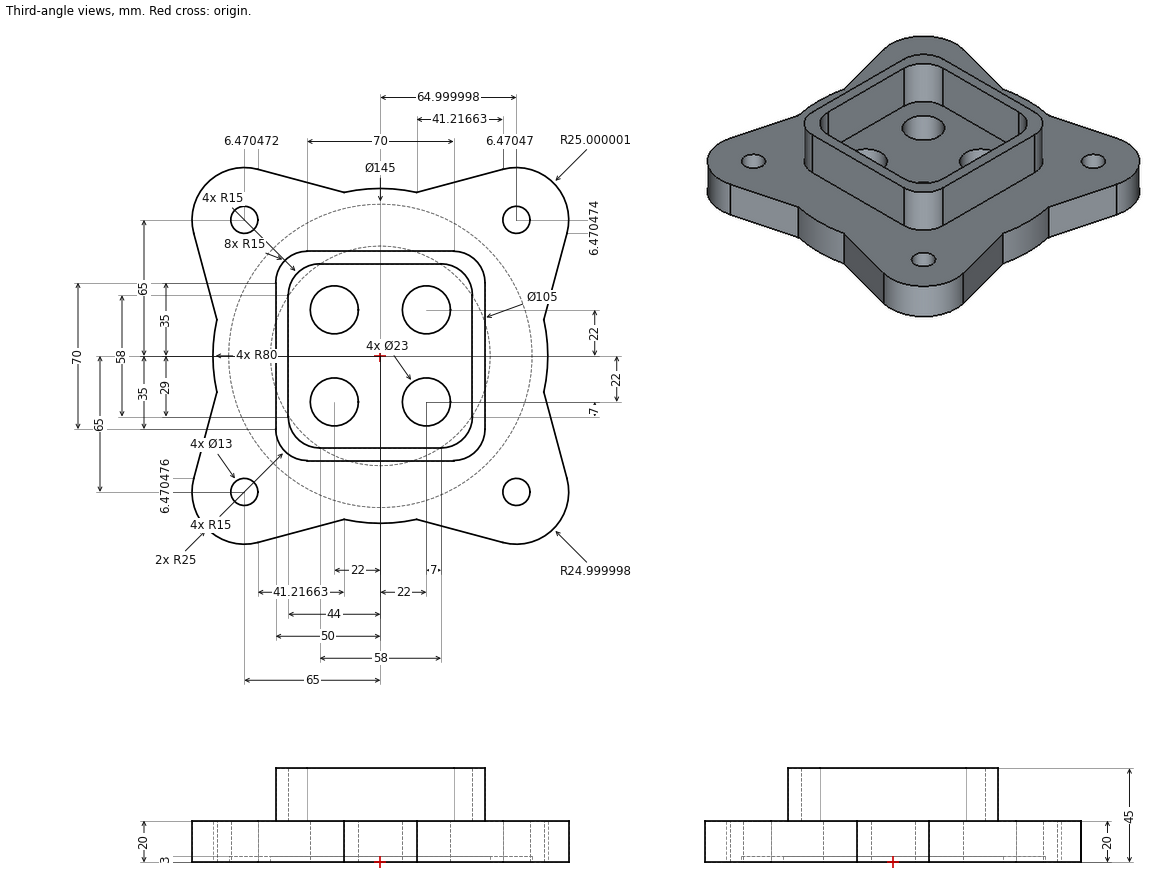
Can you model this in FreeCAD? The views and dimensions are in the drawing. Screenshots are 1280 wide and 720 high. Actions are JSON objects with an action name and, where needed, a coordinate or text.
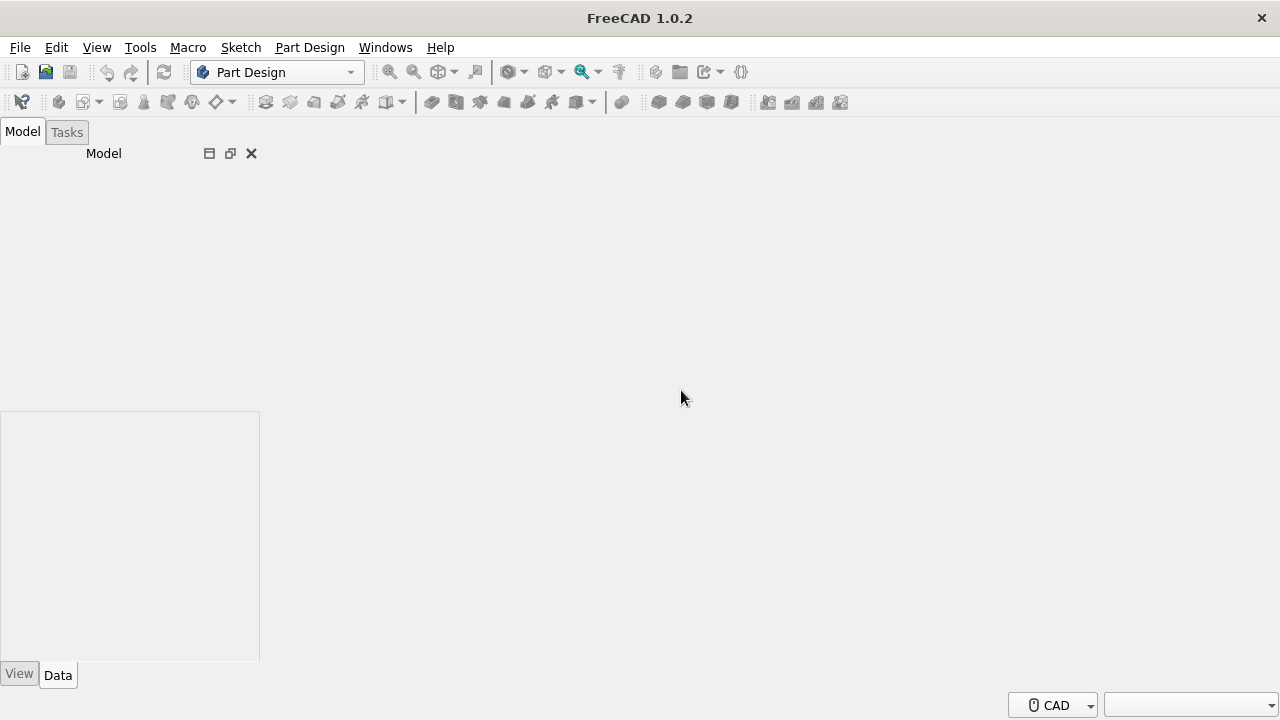
{"action": "left_click", "coordinate": [22, 72]}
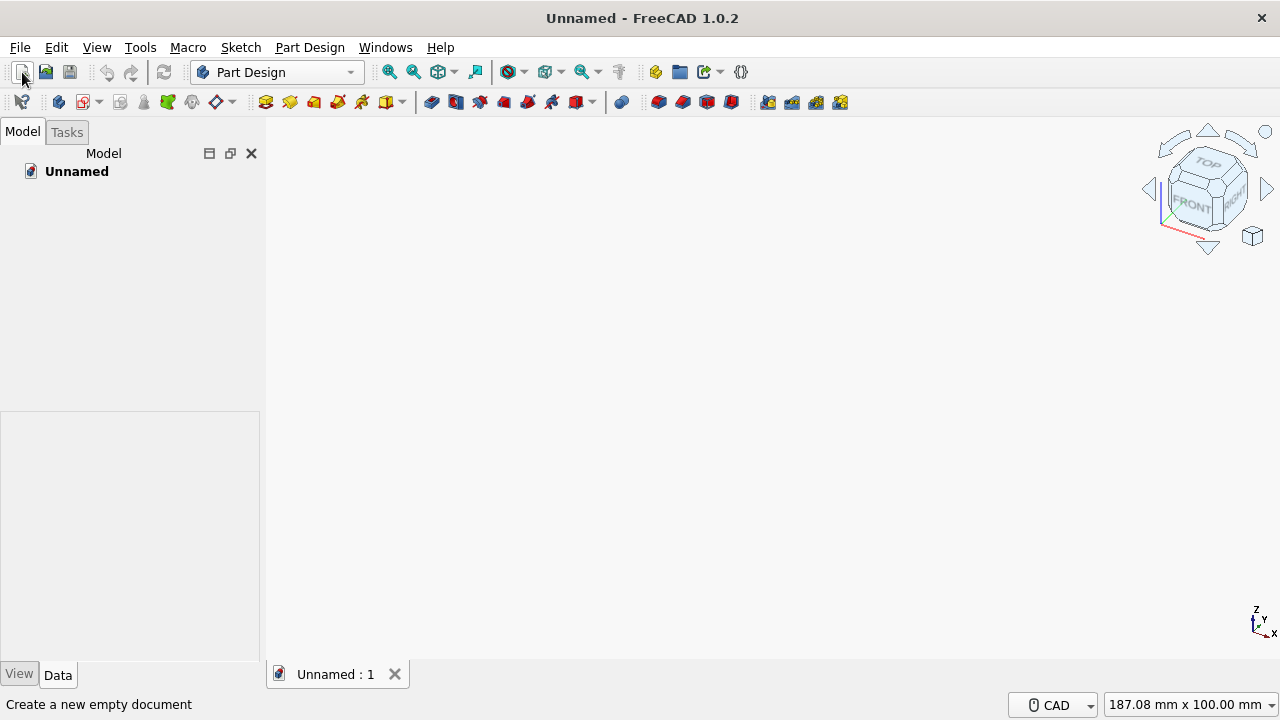
{"action": "left_click", "coordinate": [84, 102]}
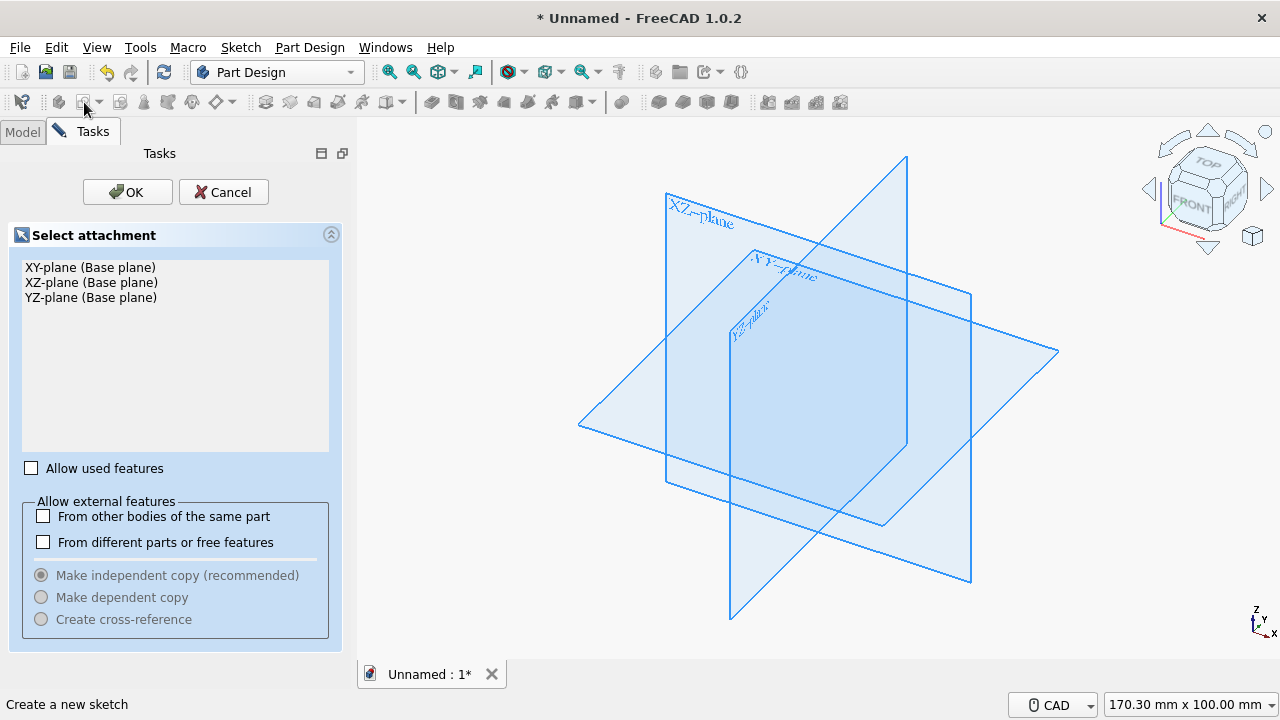
{"action": "left_click", "coordinate": [82, 268]}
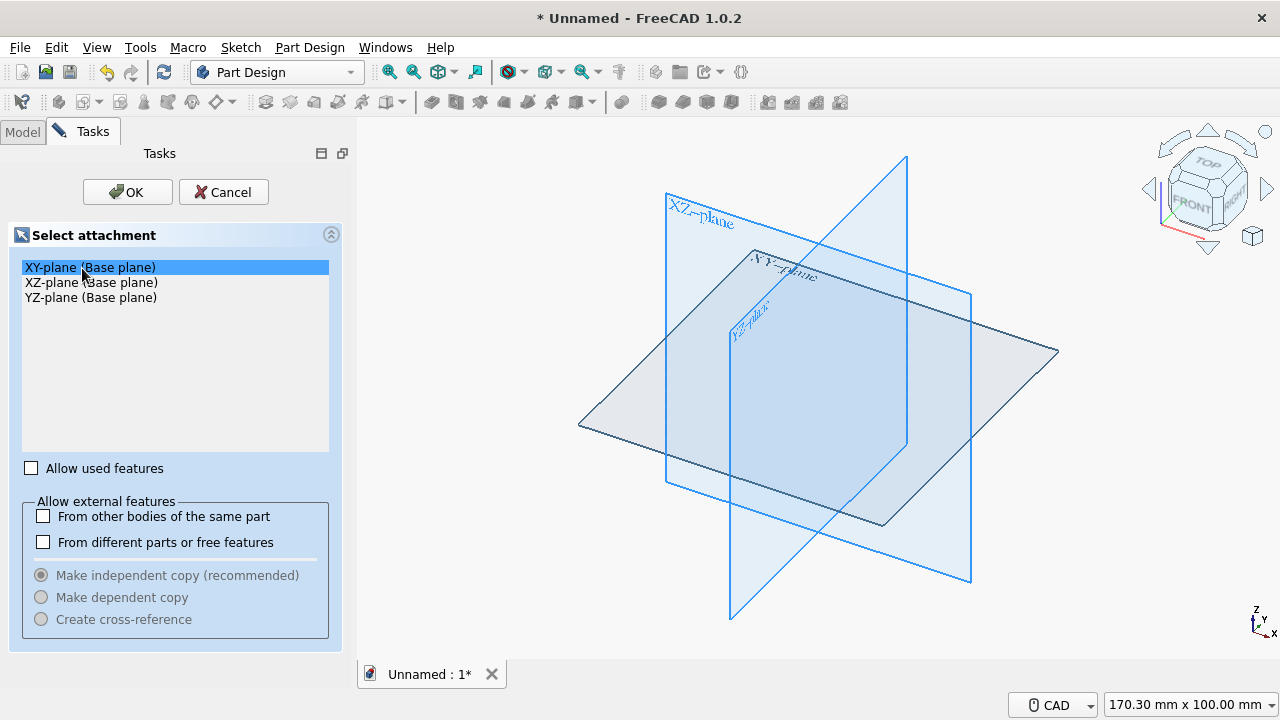
{"action": "left_click", "coordinate": [128, 192]}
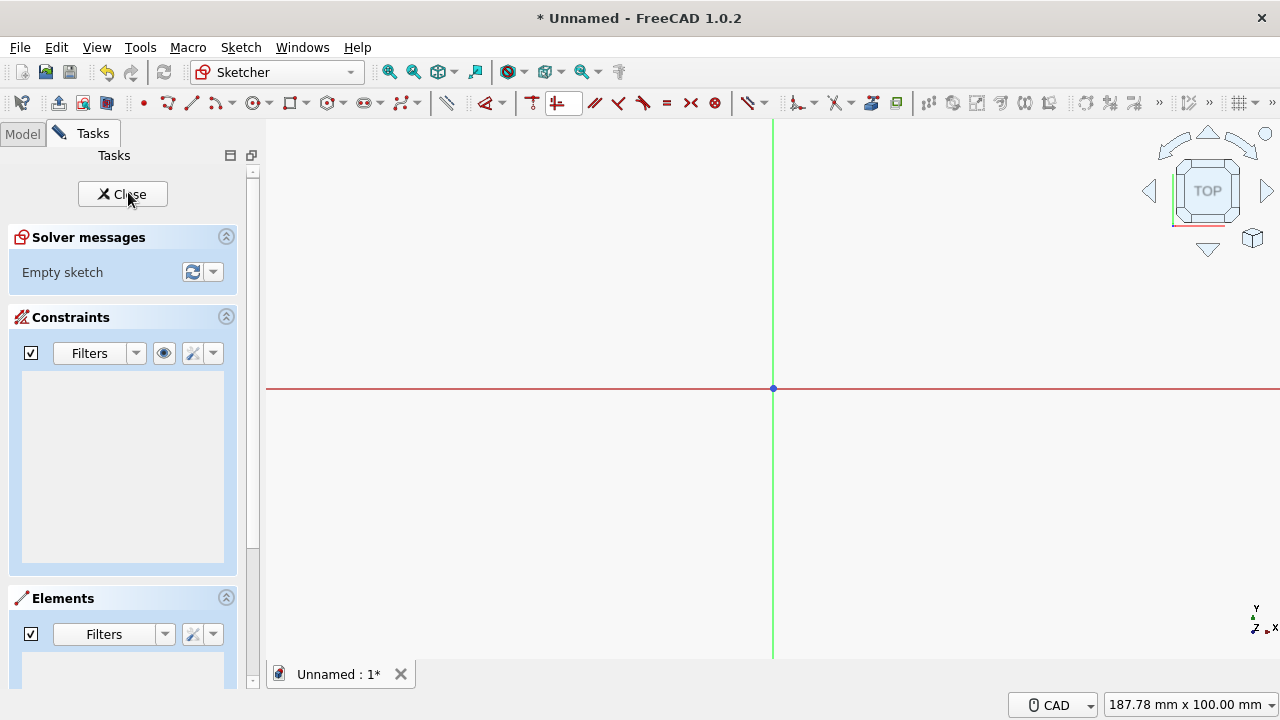
{"action": "scroll", "coordinate": [665, 389], "scroll_direction": "down", "scroll_amount": 5}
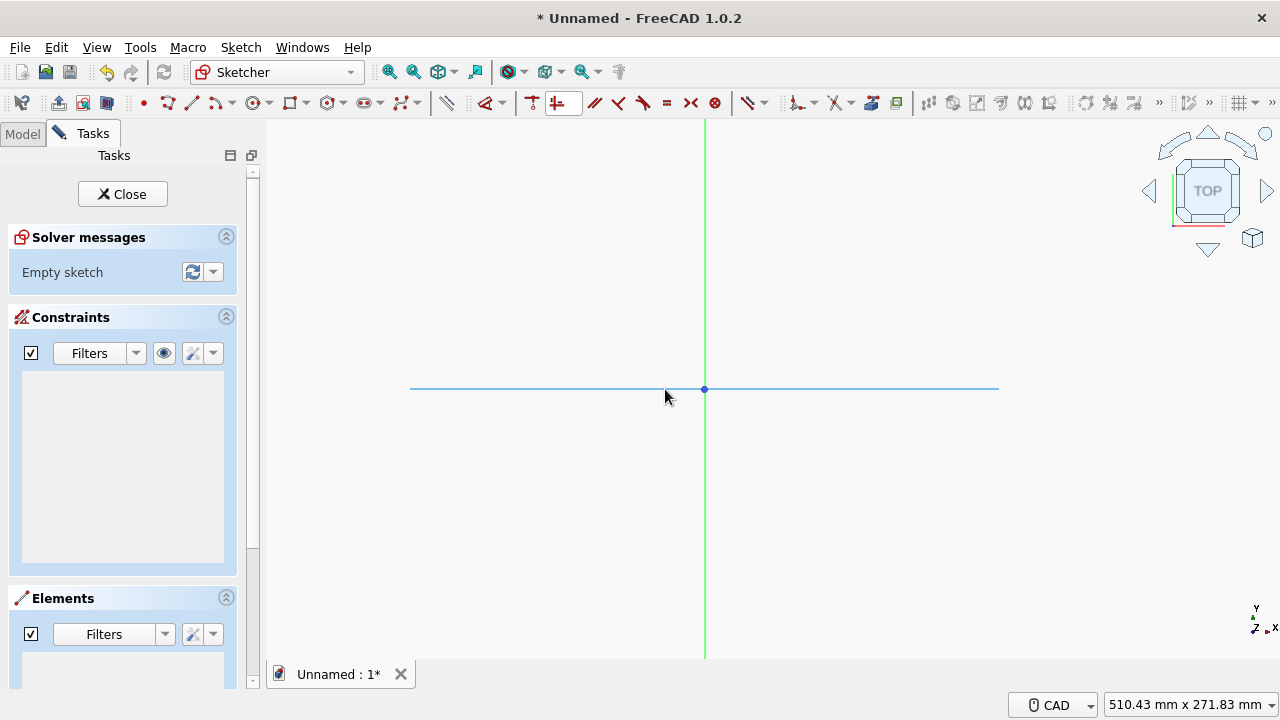
{"action": "left_click", "coordinate": [192, 104]}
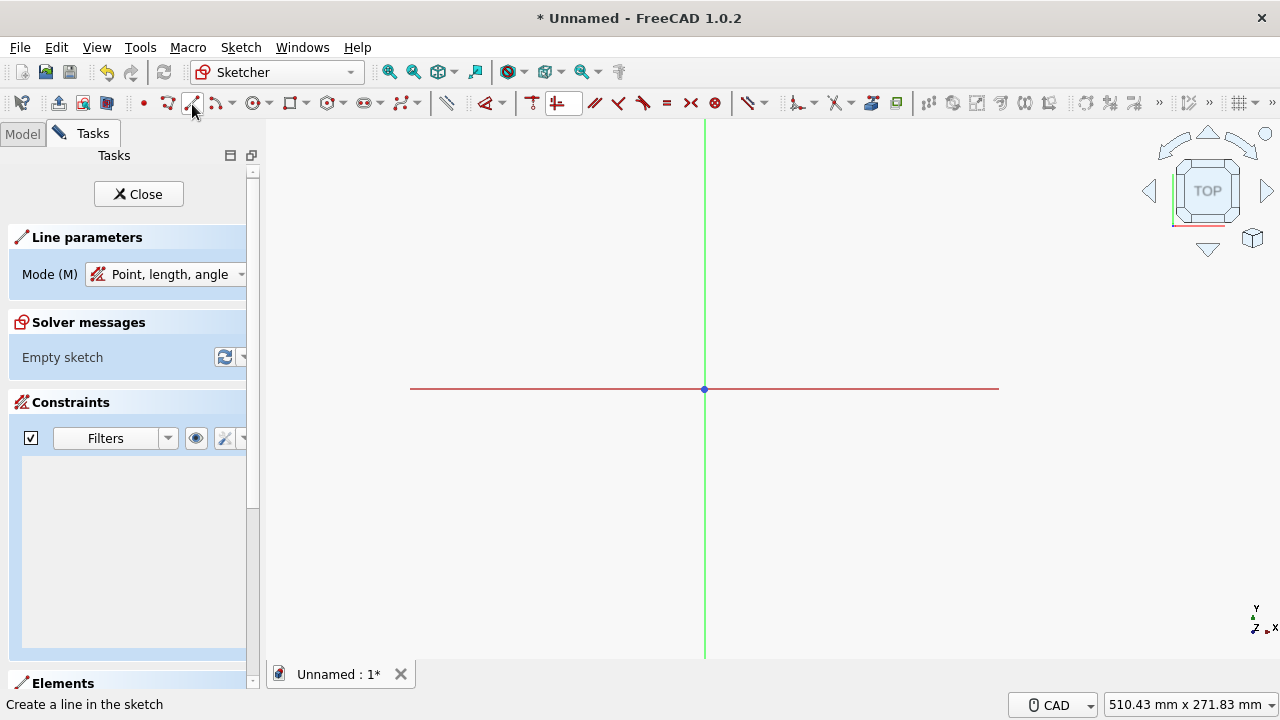
{"action": "left_click", "coordinate": [528, 273]}
{"action": "left_click", "coordinate": [550, 355]}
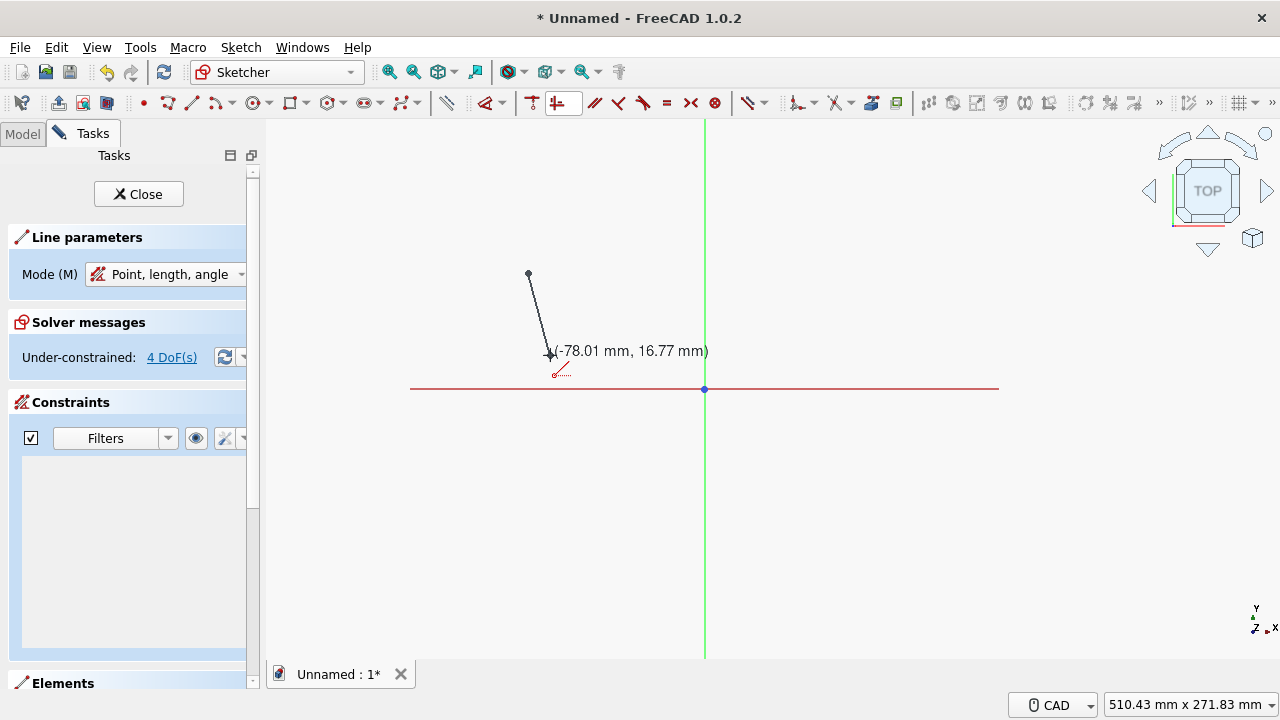
{"action": "left_click", "coordinate": [550, 424]}
{"action": "left_click", "coordinate": [528, 506]}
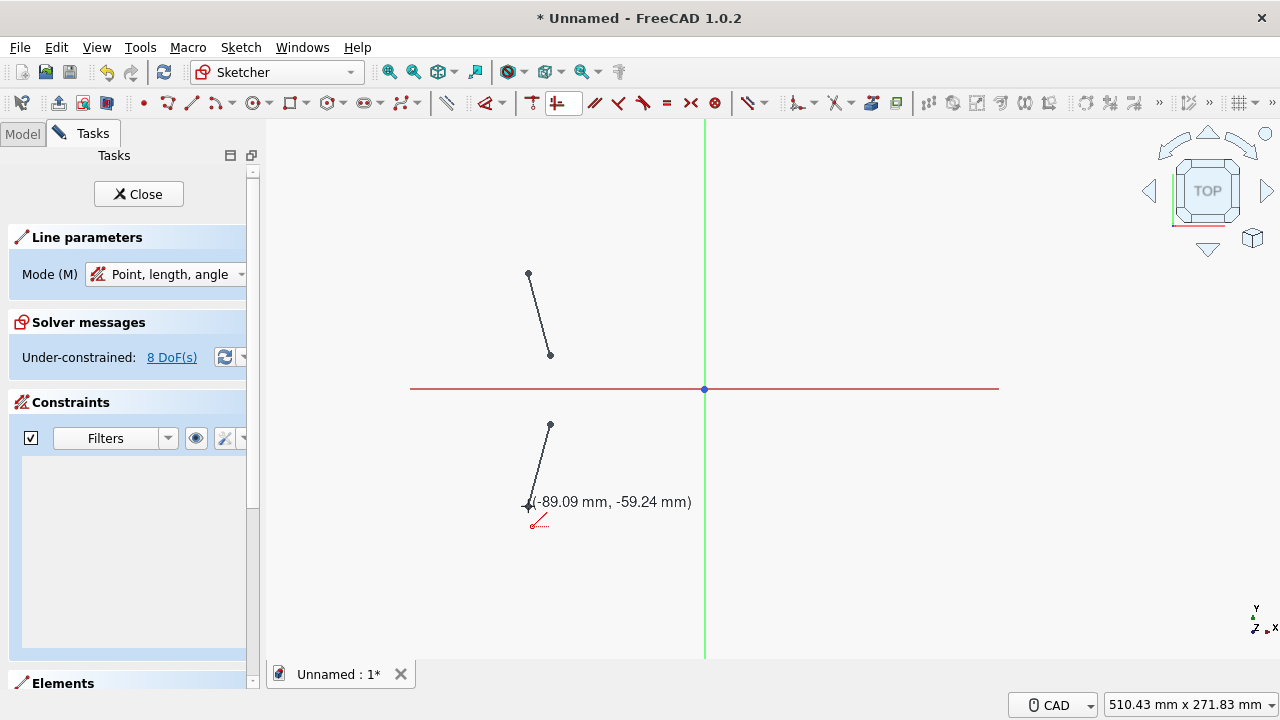
{"action": "left_click", "coordinate": [589, 566]}
{"action": "left_click", "coordinate": [671, 544]}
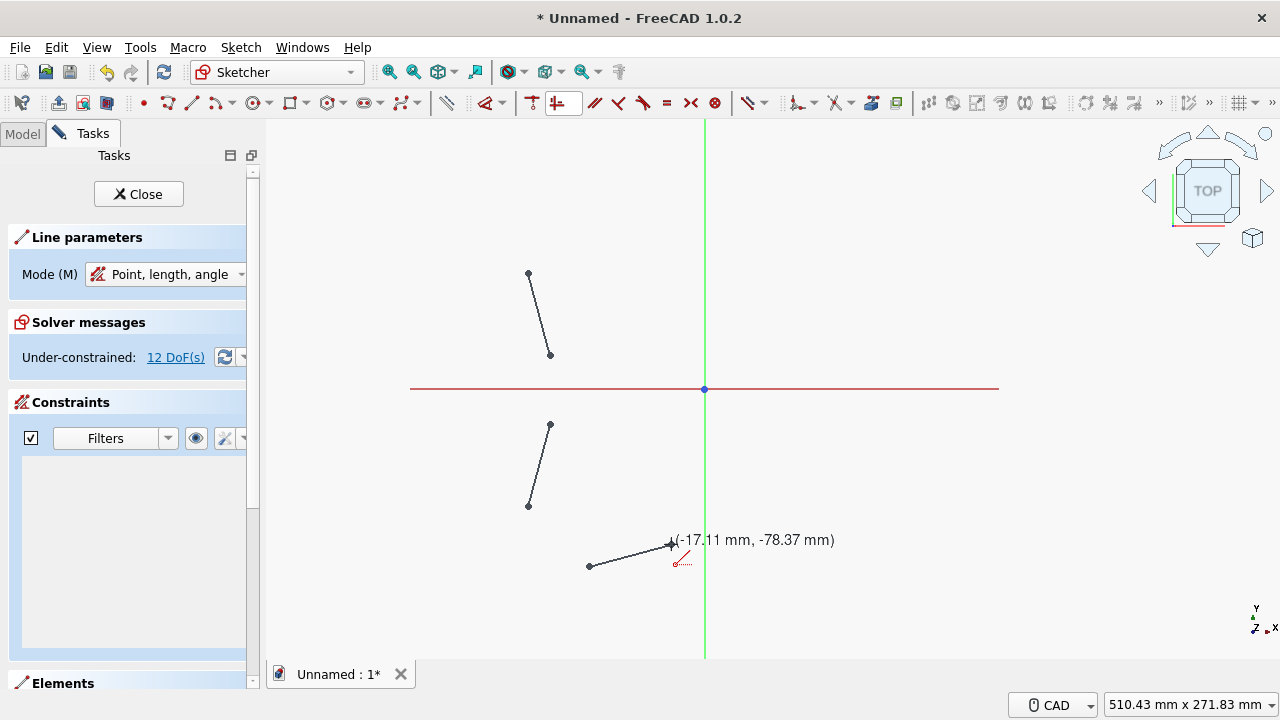
{"action": "left_click", "coordinate": [739, 544]}
{"action": "left_click", "coordinate": [821, 566]}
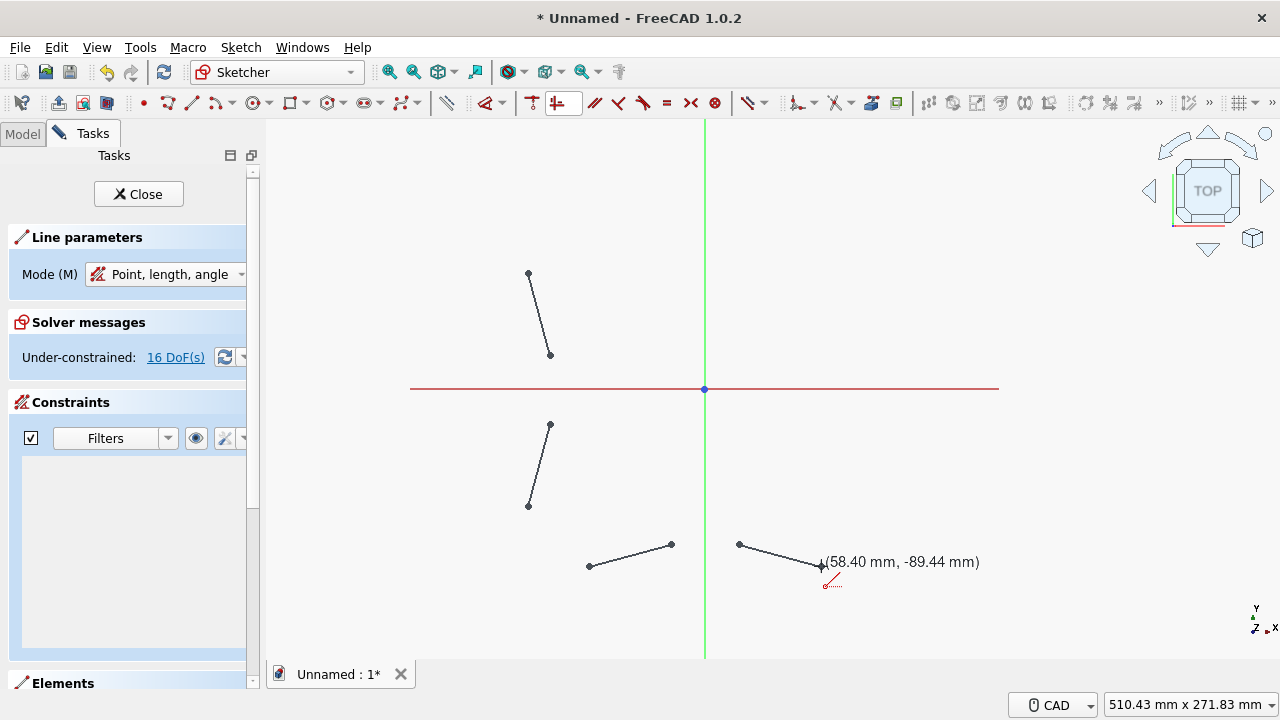
{"action": "left_click", "coordinate": [882, 506]}
{"action": "left_click", "coordinate": [860, 424]}